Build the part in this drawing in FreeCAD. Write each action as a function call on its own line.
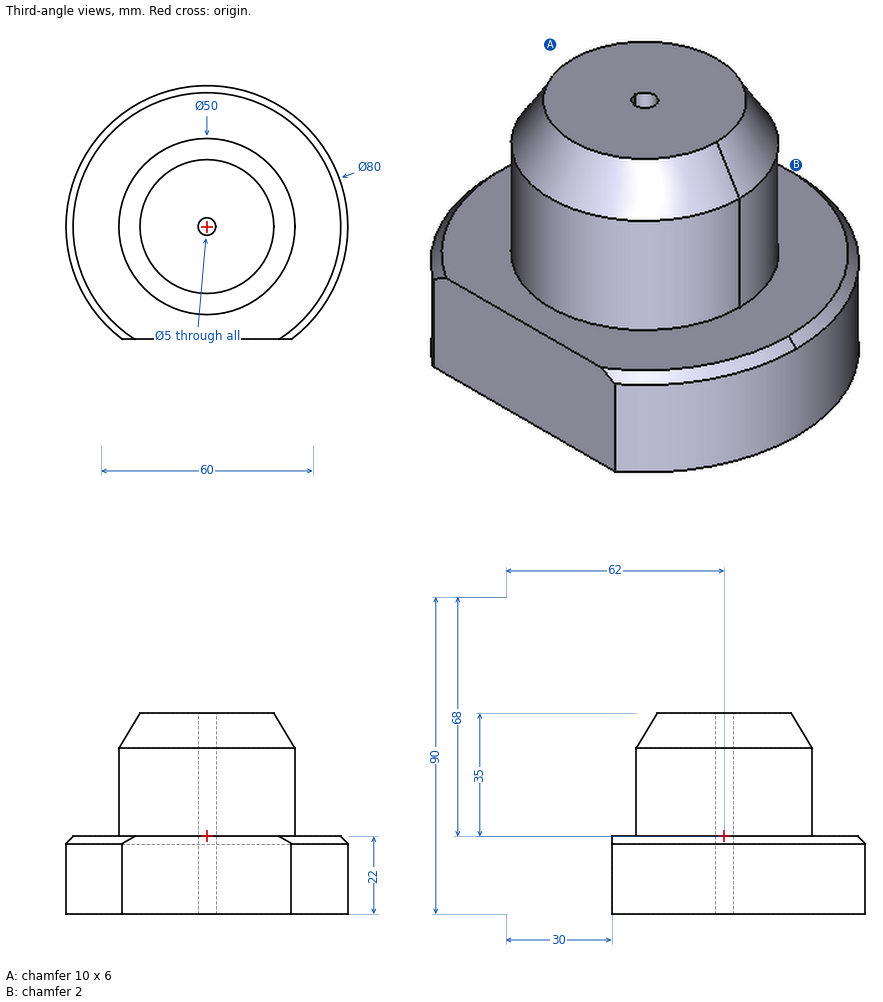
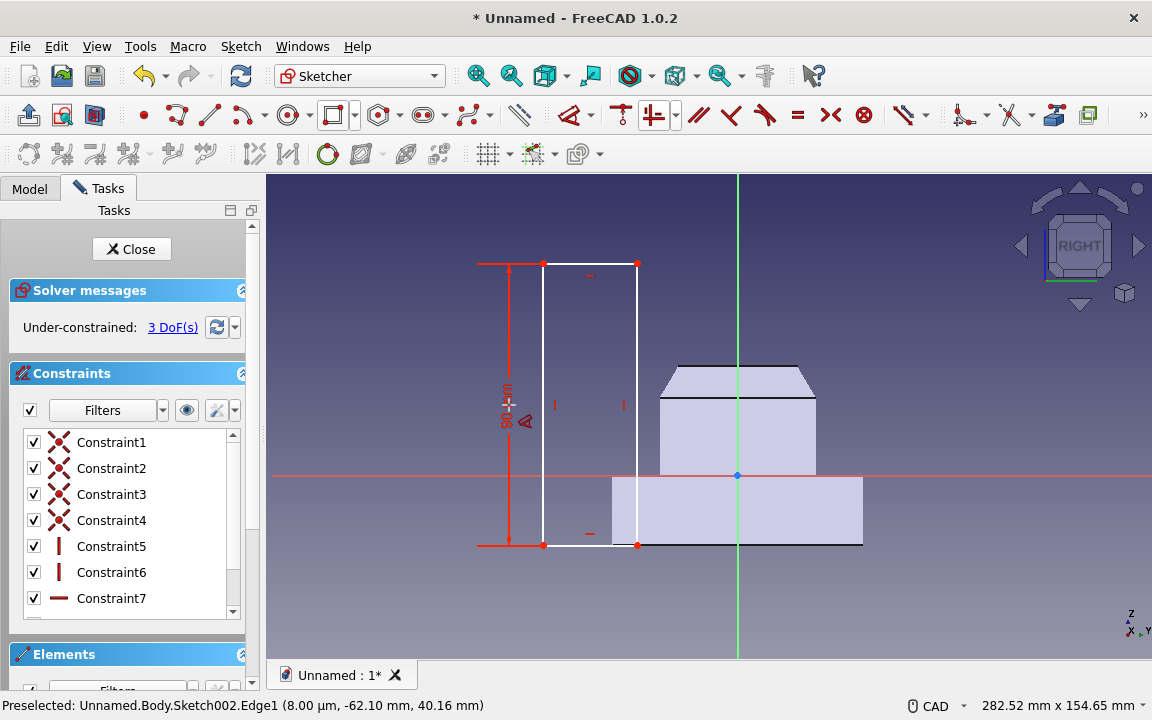
click(571, 546)
click(590, 580)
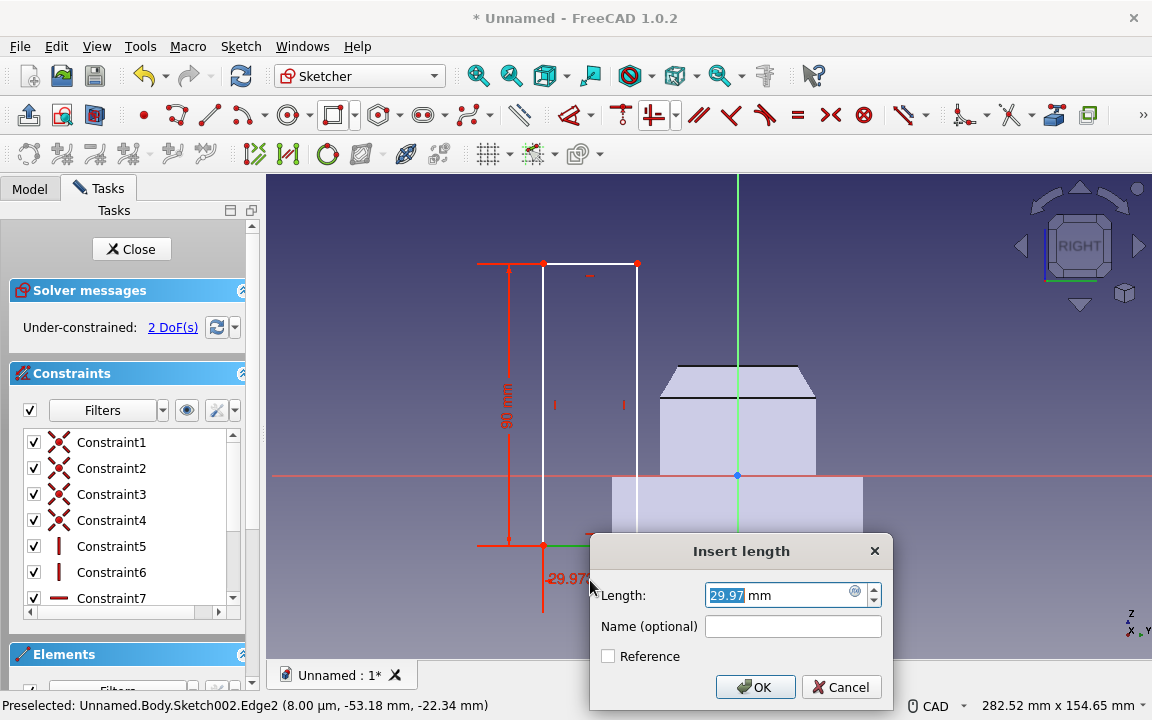
text(30)
key(Return)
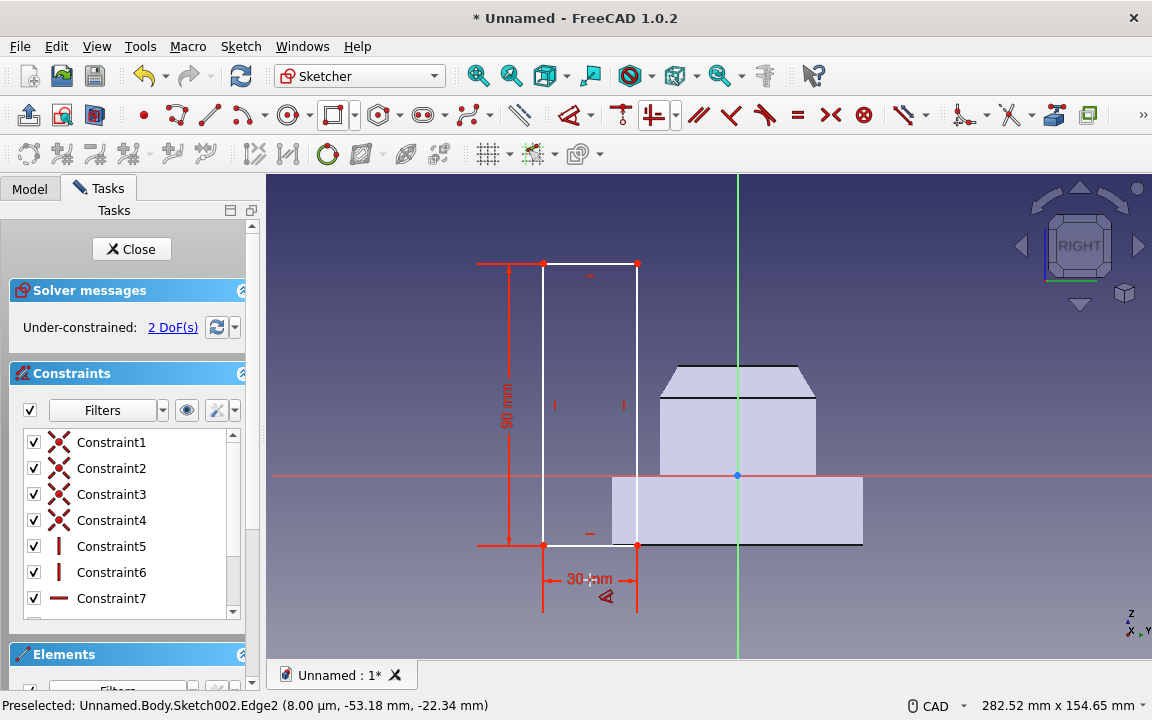
click(543, 264)
click(640, 230)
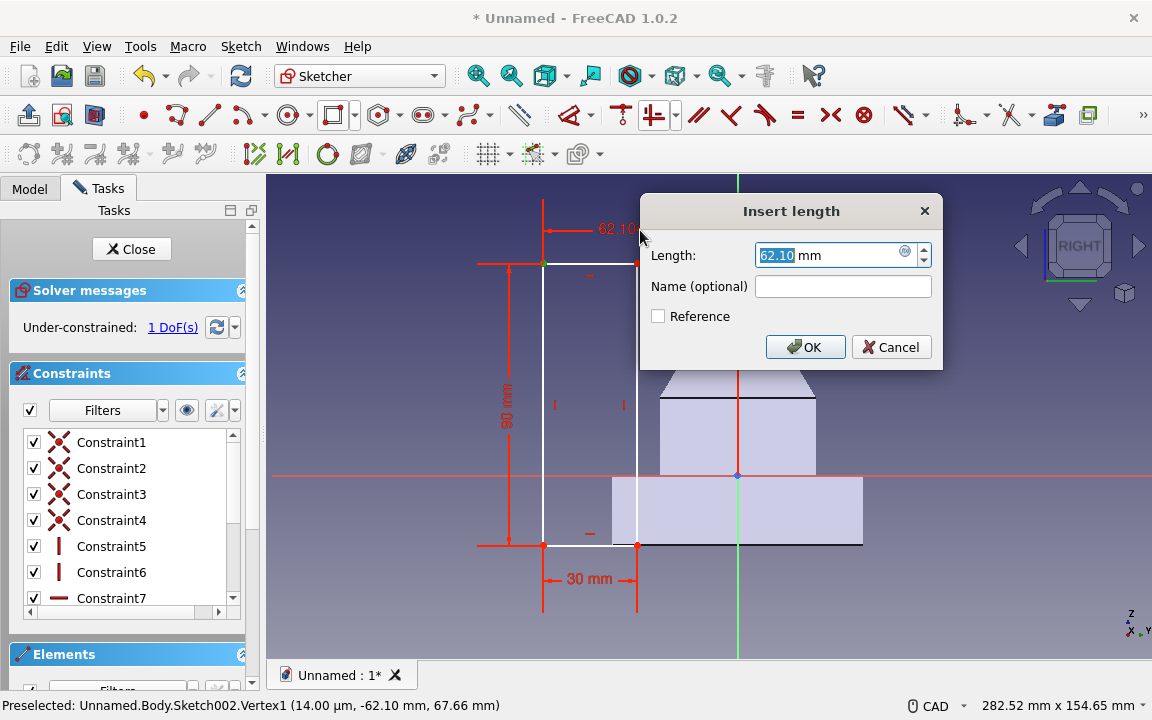
text(62)
key(Return)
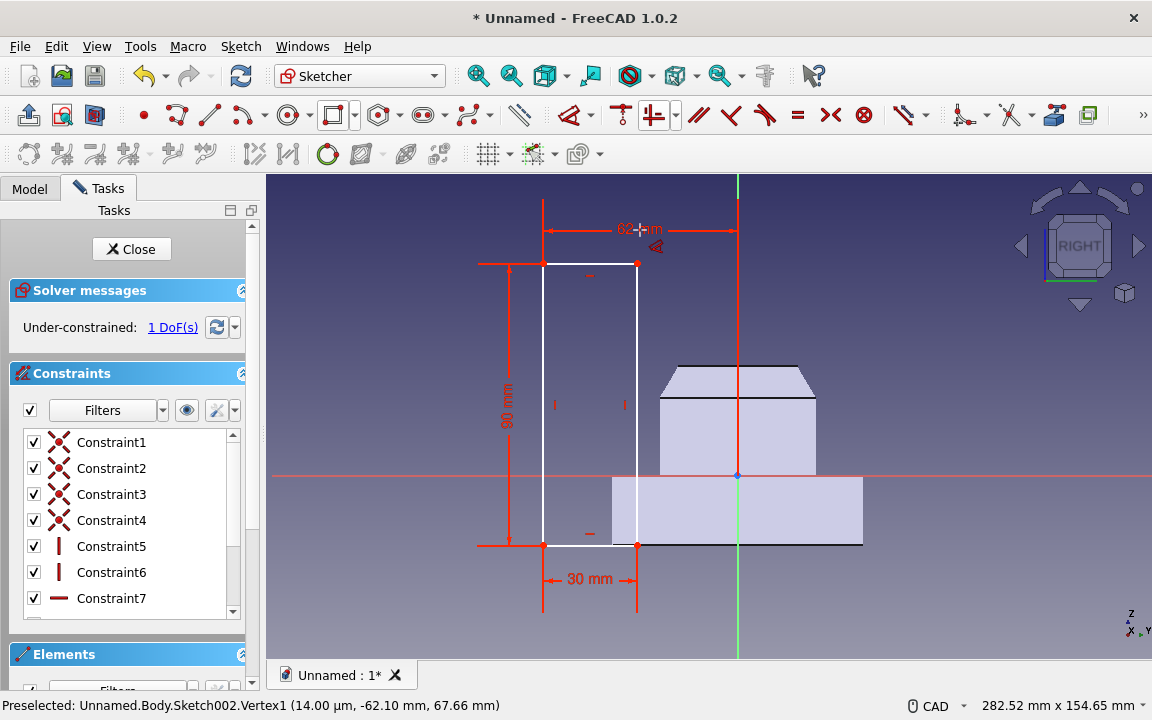
click(543, 264)
click(772, 370)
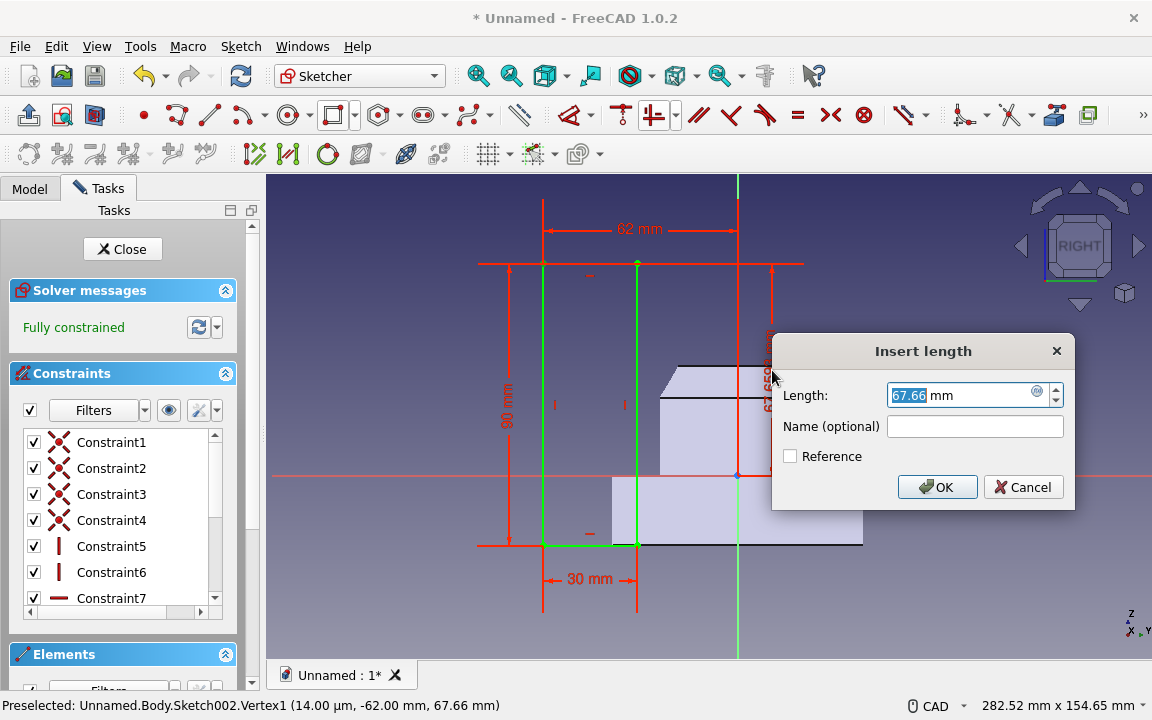
text(68)
key(Return)
key(Escape)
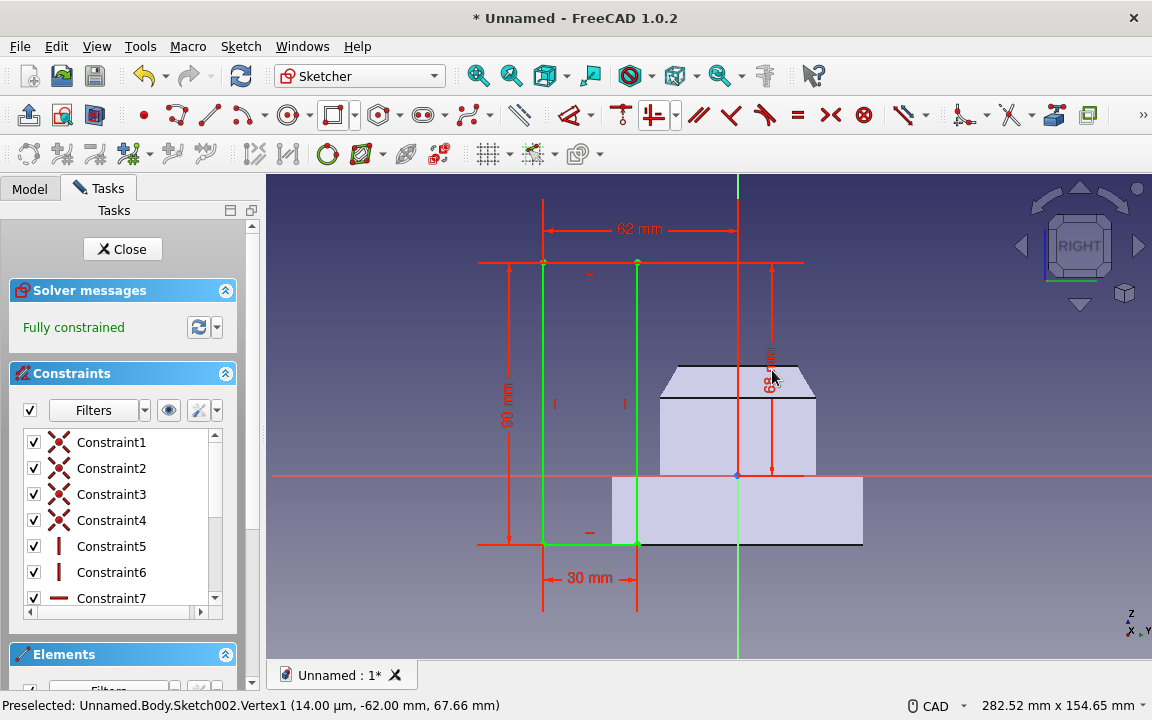
click(123, 249)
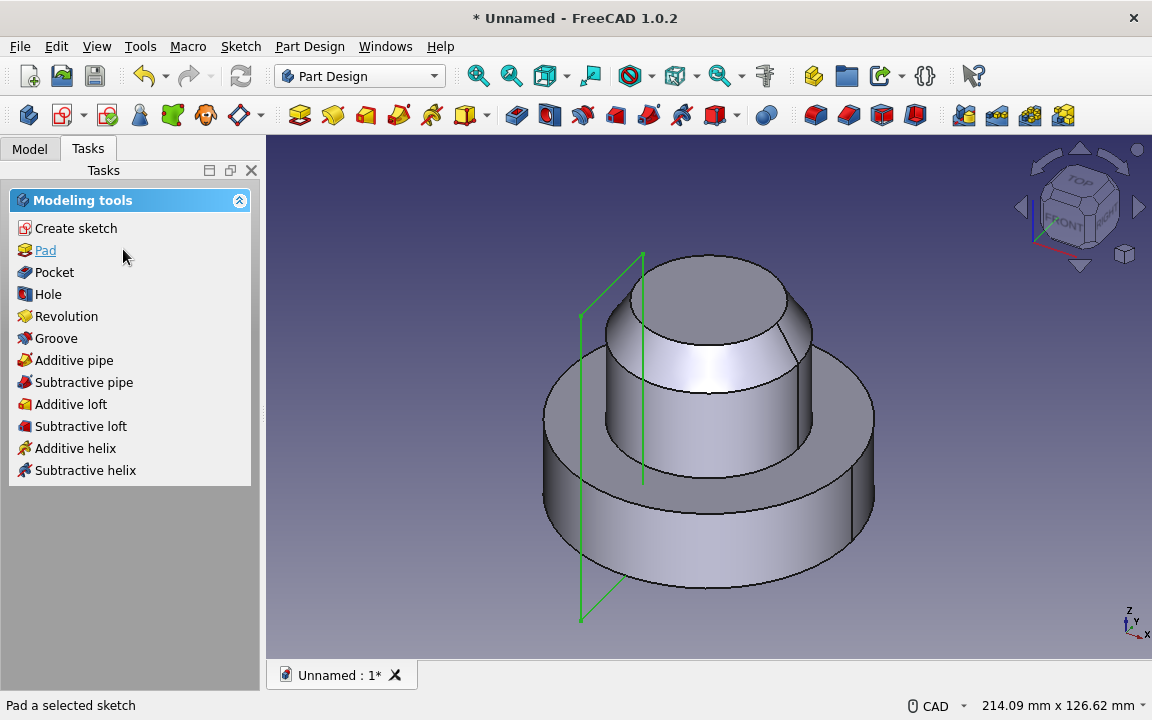
click(517, 116)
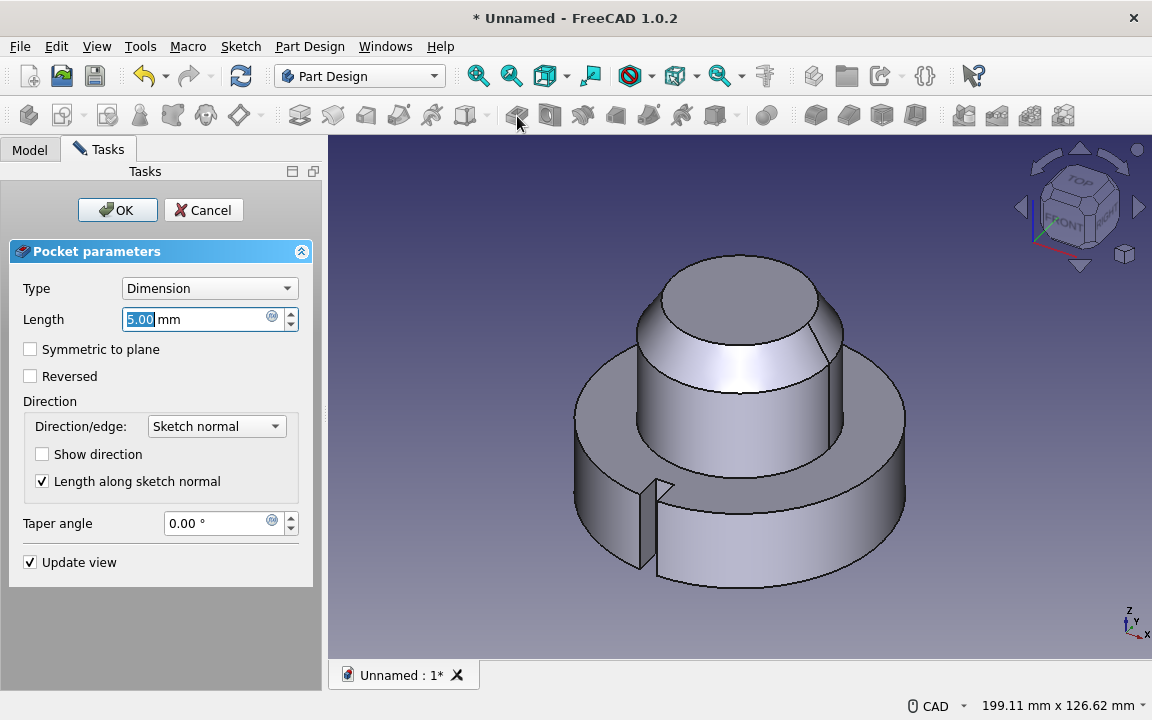
text(60)
key(Tab)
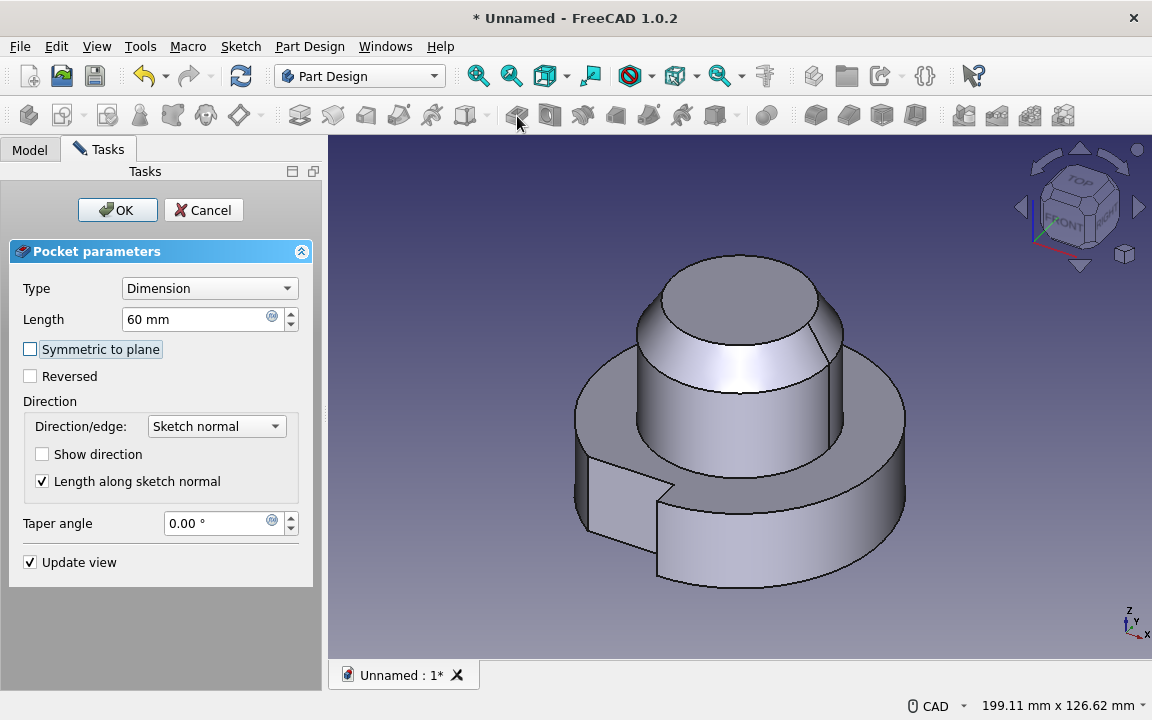
click(31, 349)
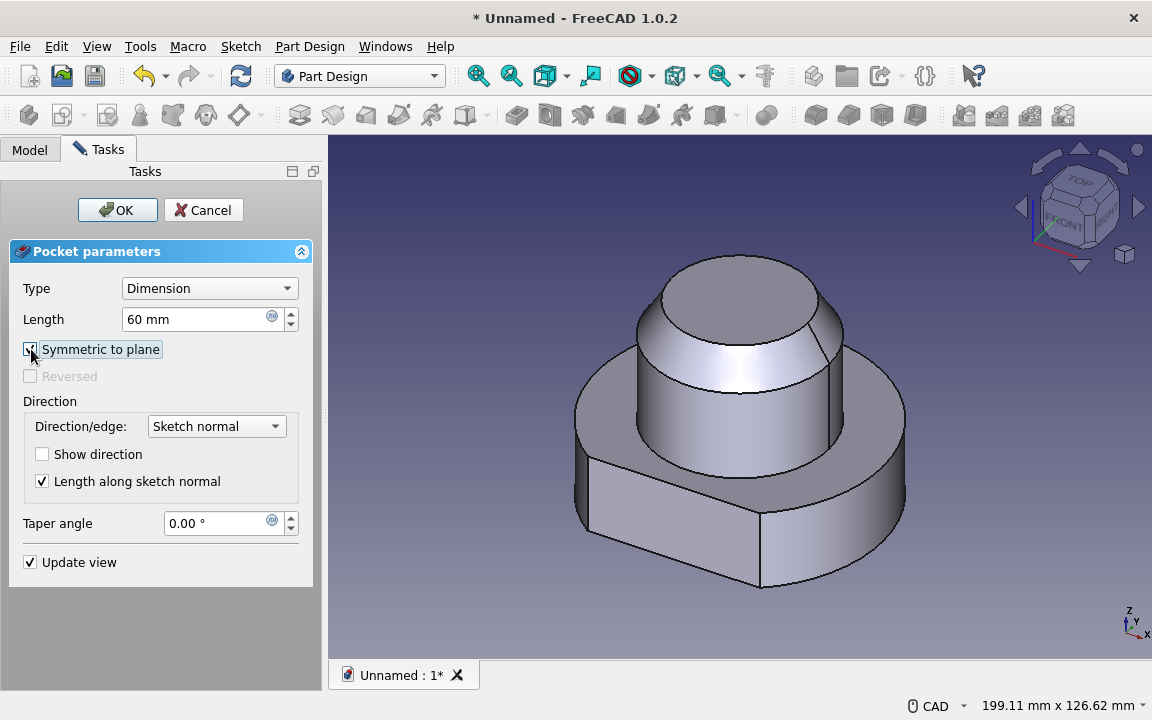
click(118, 210)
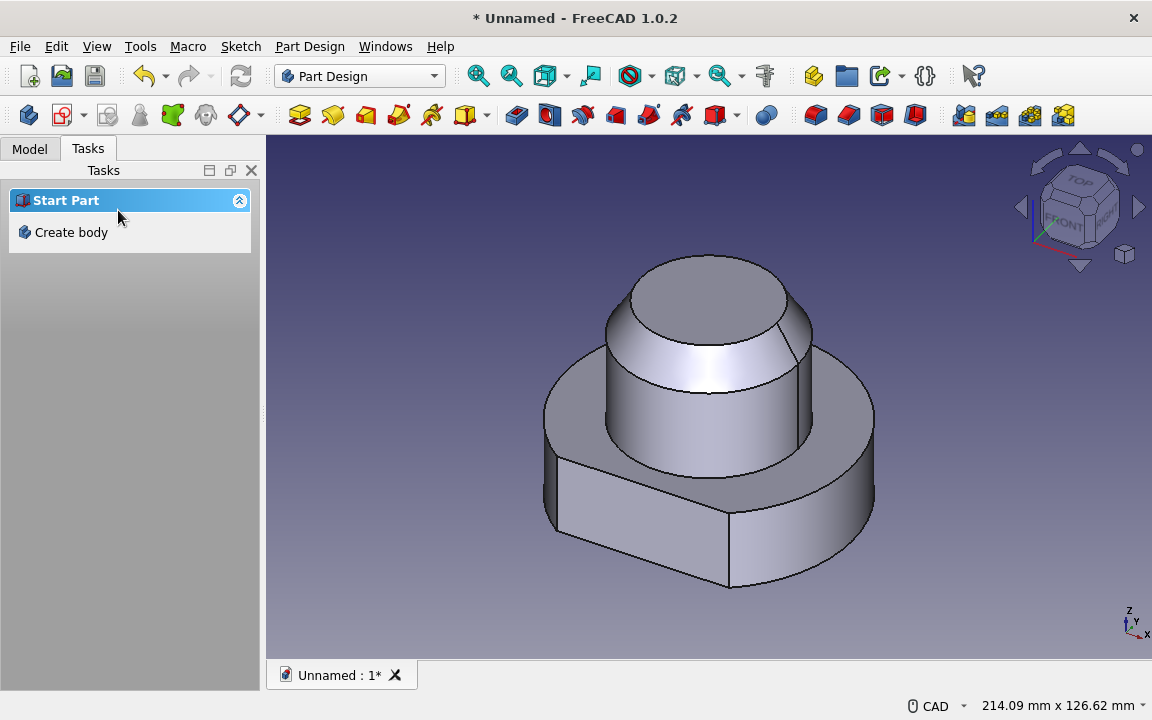
click(874, 421)